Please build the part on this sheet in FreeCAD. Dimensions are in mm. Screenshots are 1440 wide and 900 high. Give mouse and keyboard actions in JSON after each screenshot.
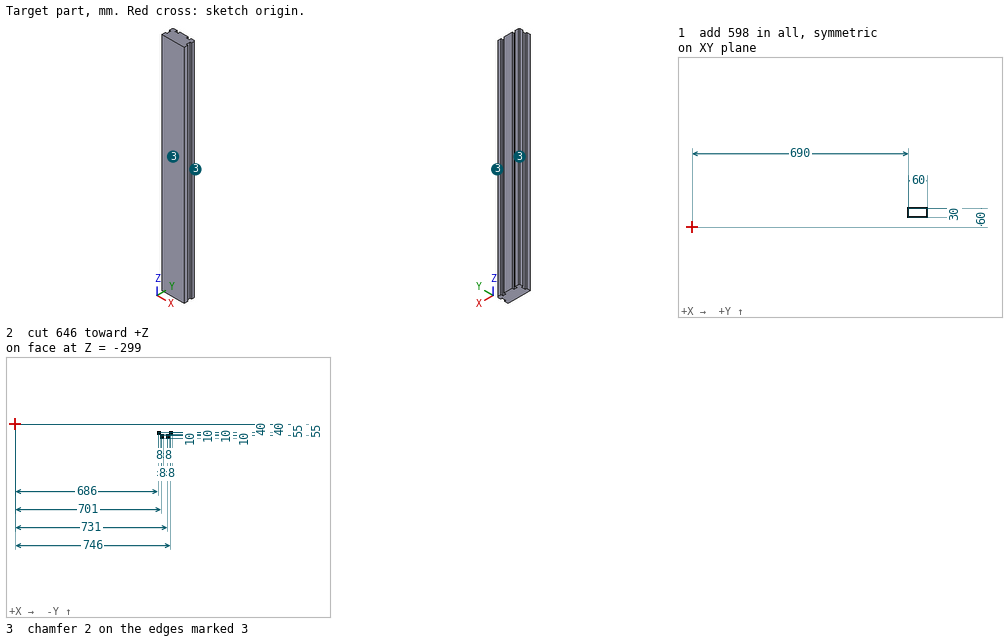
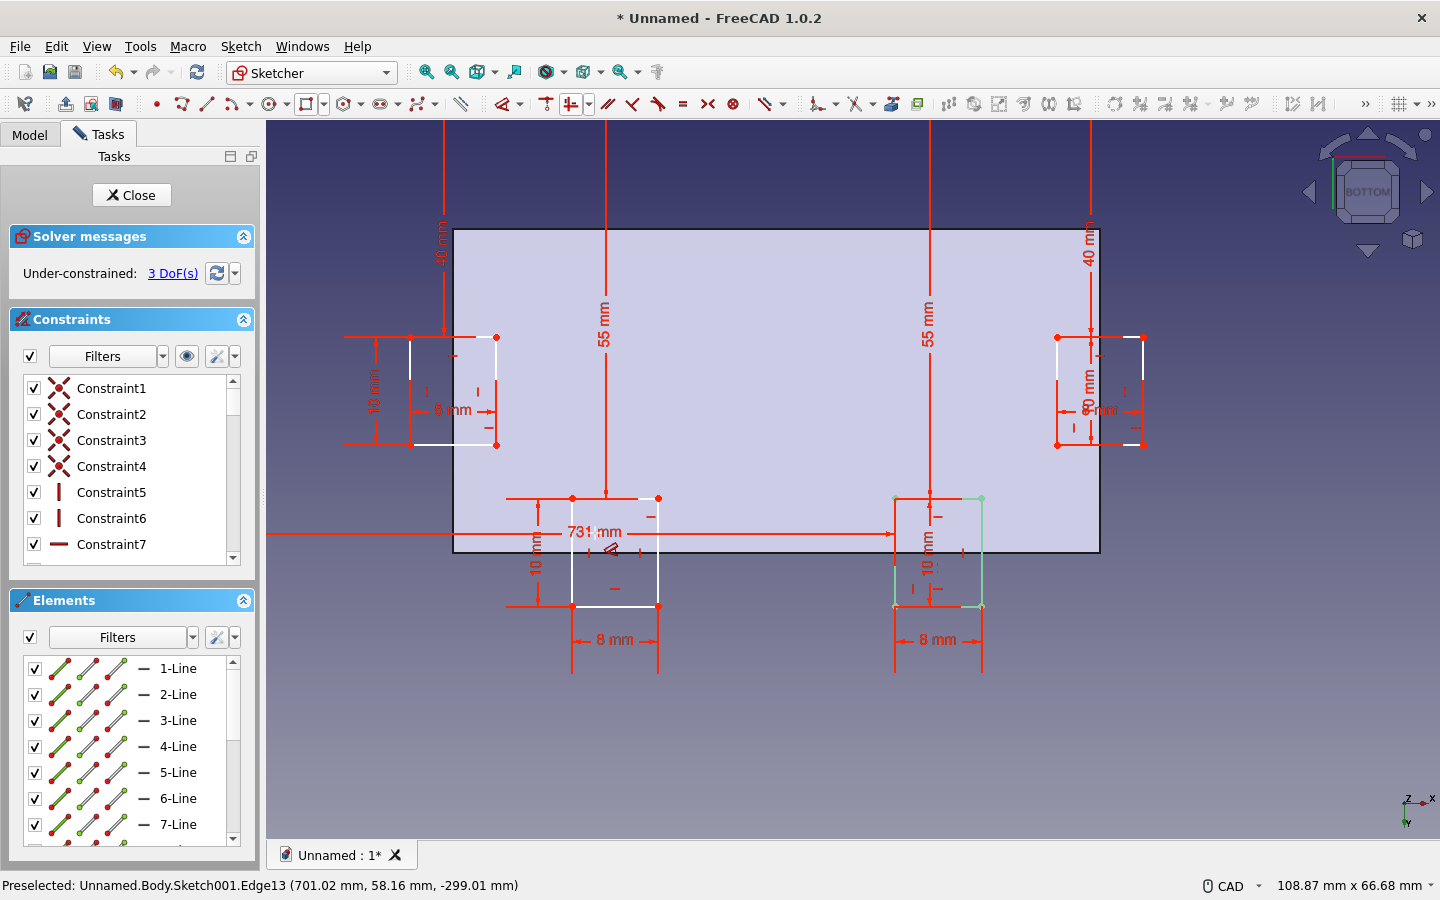
{"action": "left_click", "coordinate": [1057, 337]}
{"action": "left_click", "coordinate": [676, 371]}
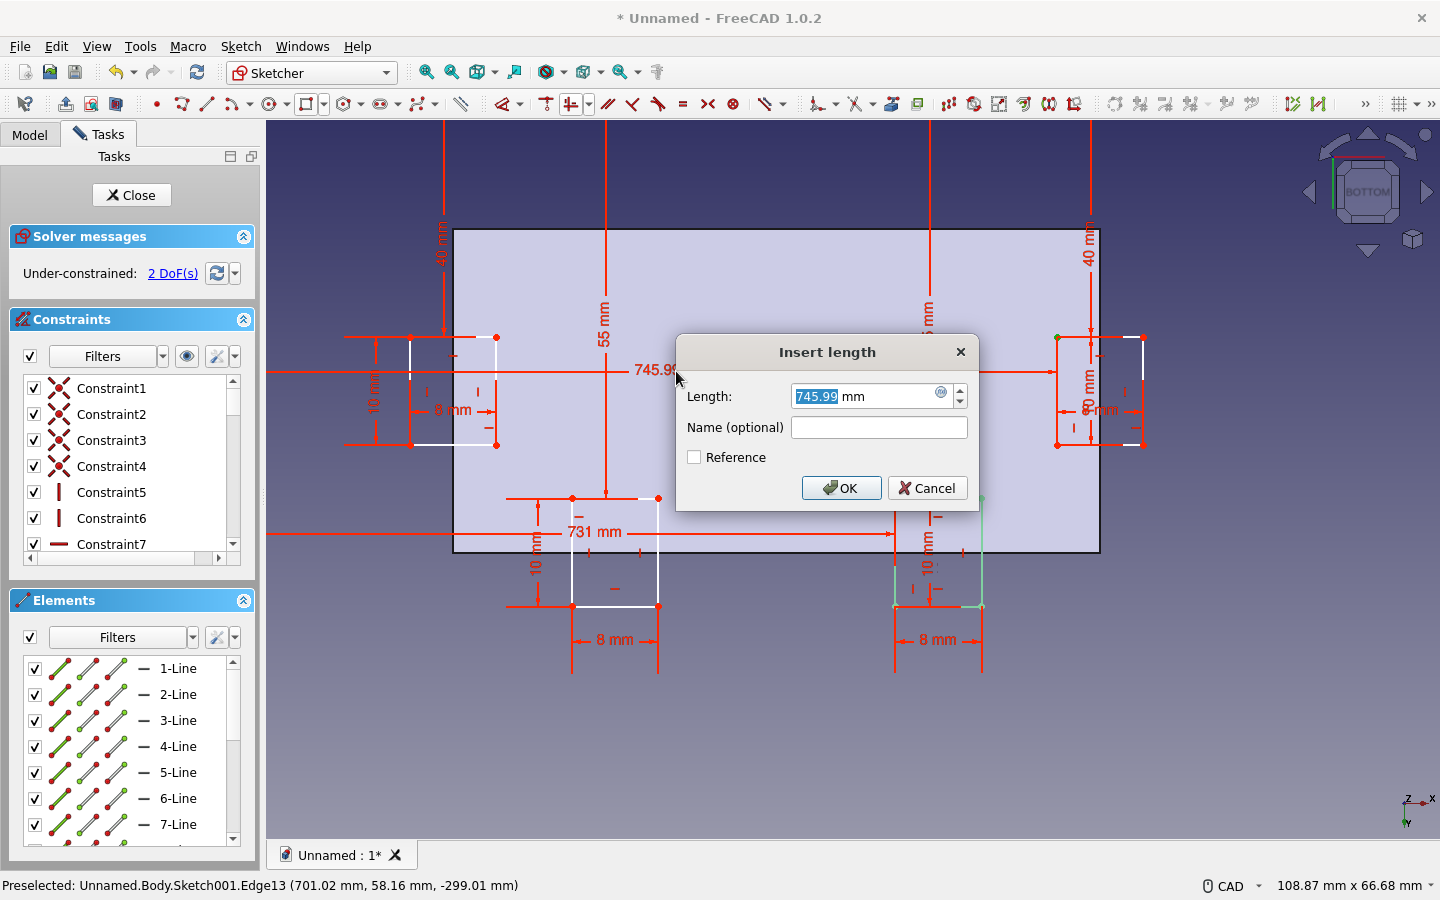
{"action": "type", "text": "746"}
{"action": "key", "text": "Return"}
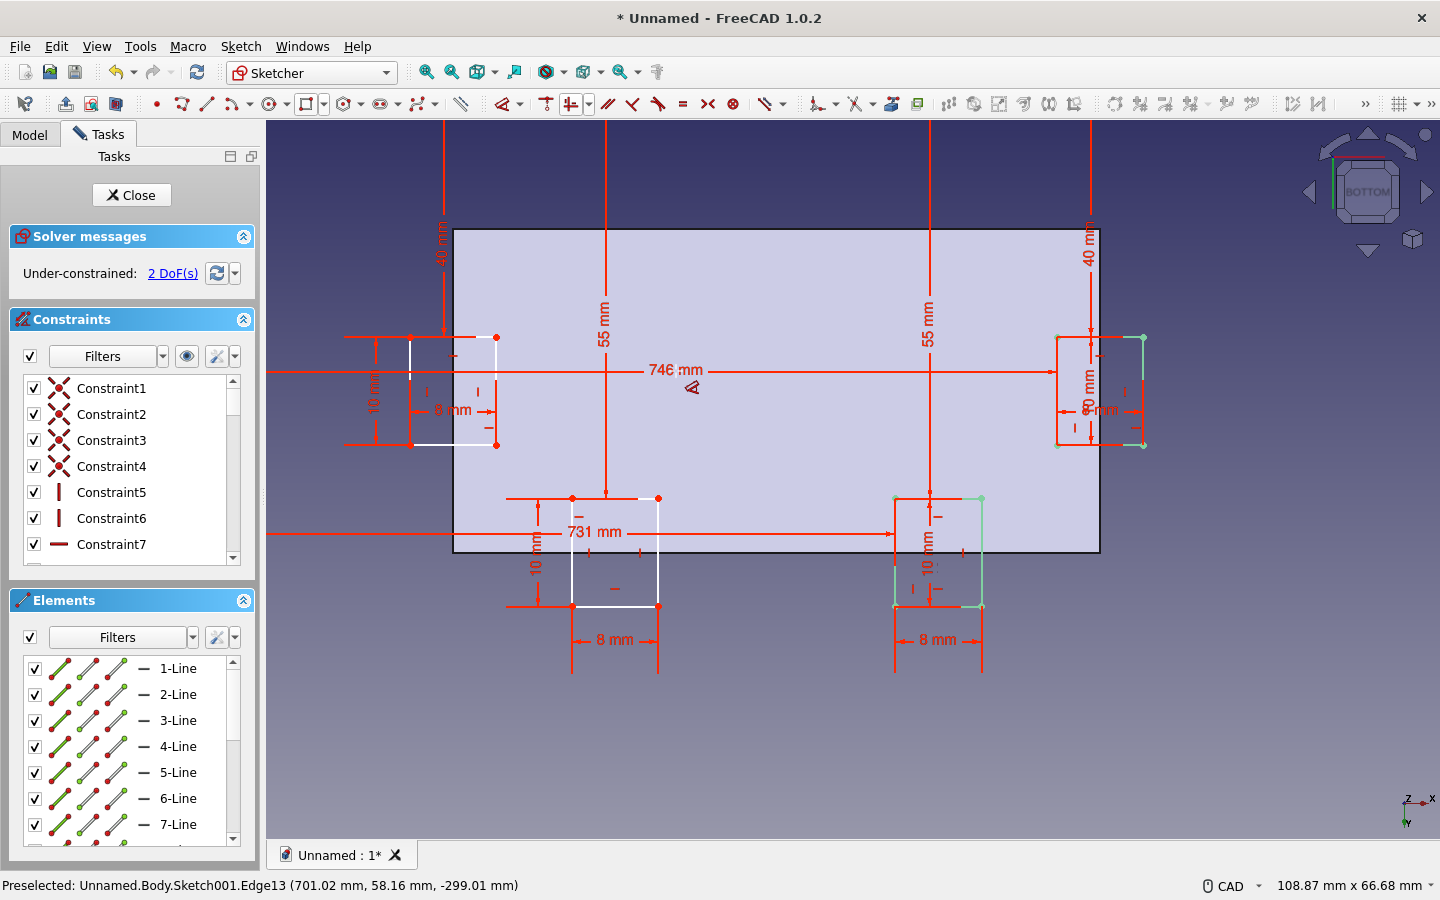
{"action": "left_click", "coordinate": [410, 337]}
{"action": "left_click", "coordinate": [352, 371]}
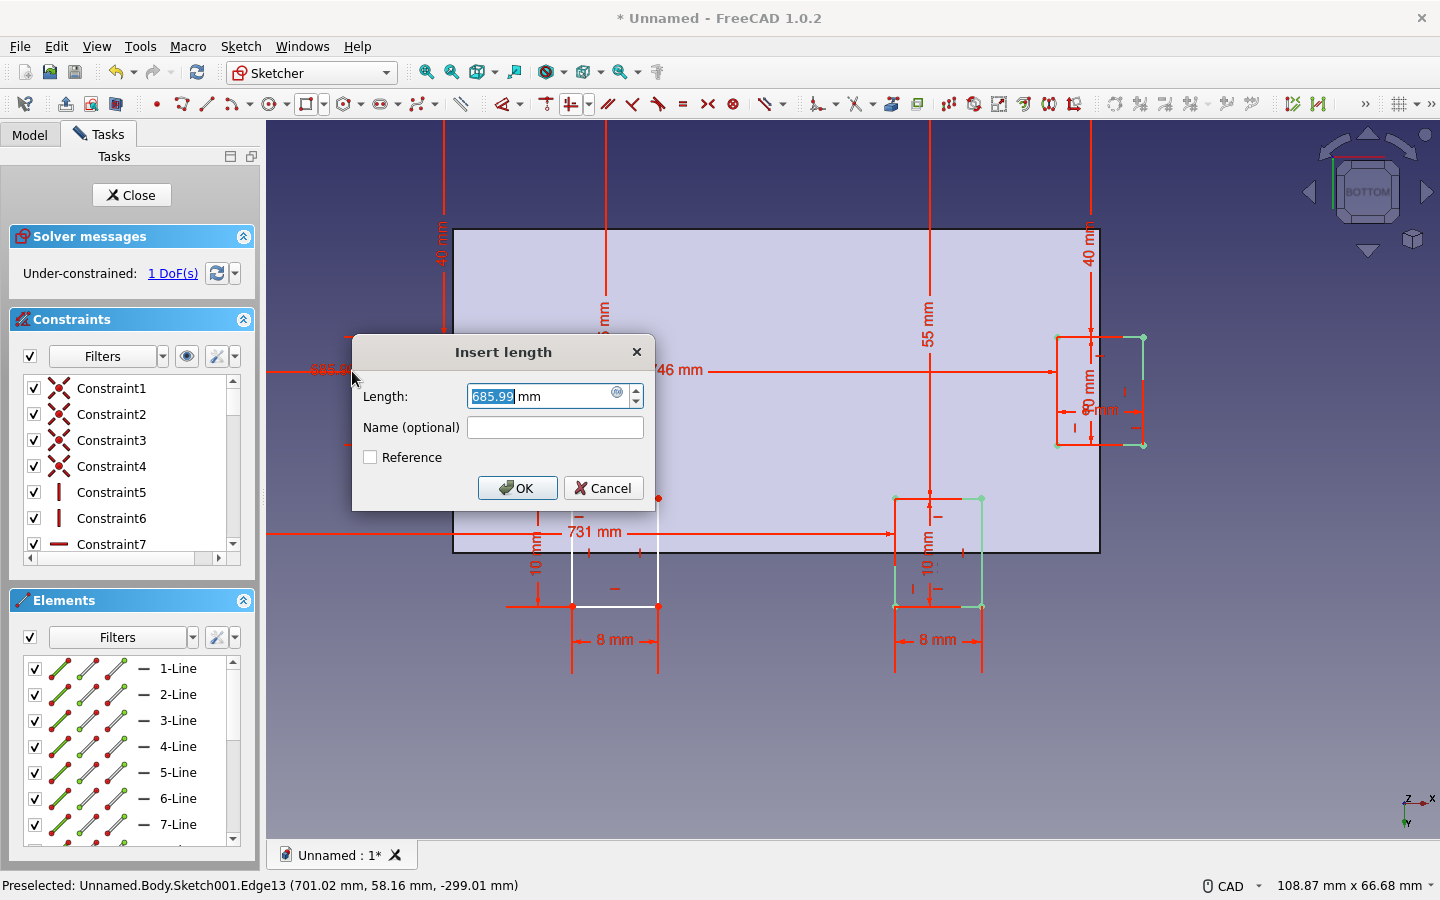
{"action": "type", "text": "686"}
{"action": "key", "text": "Return"}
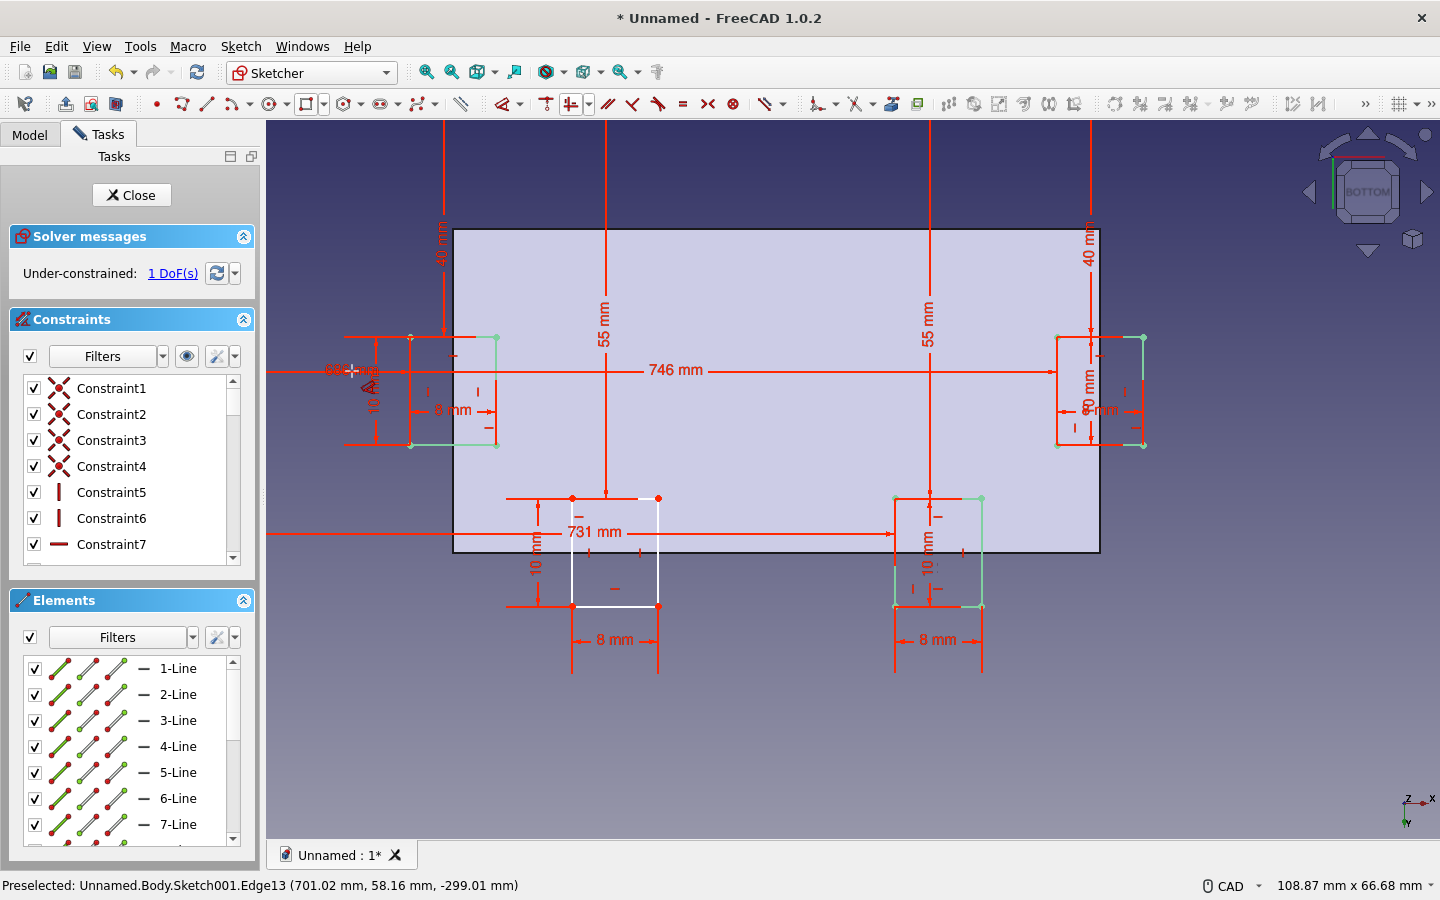
{"action": "left_click", "coordinate": [572, 499]}
{"action": "left_click", "coordinate": [433, 533]}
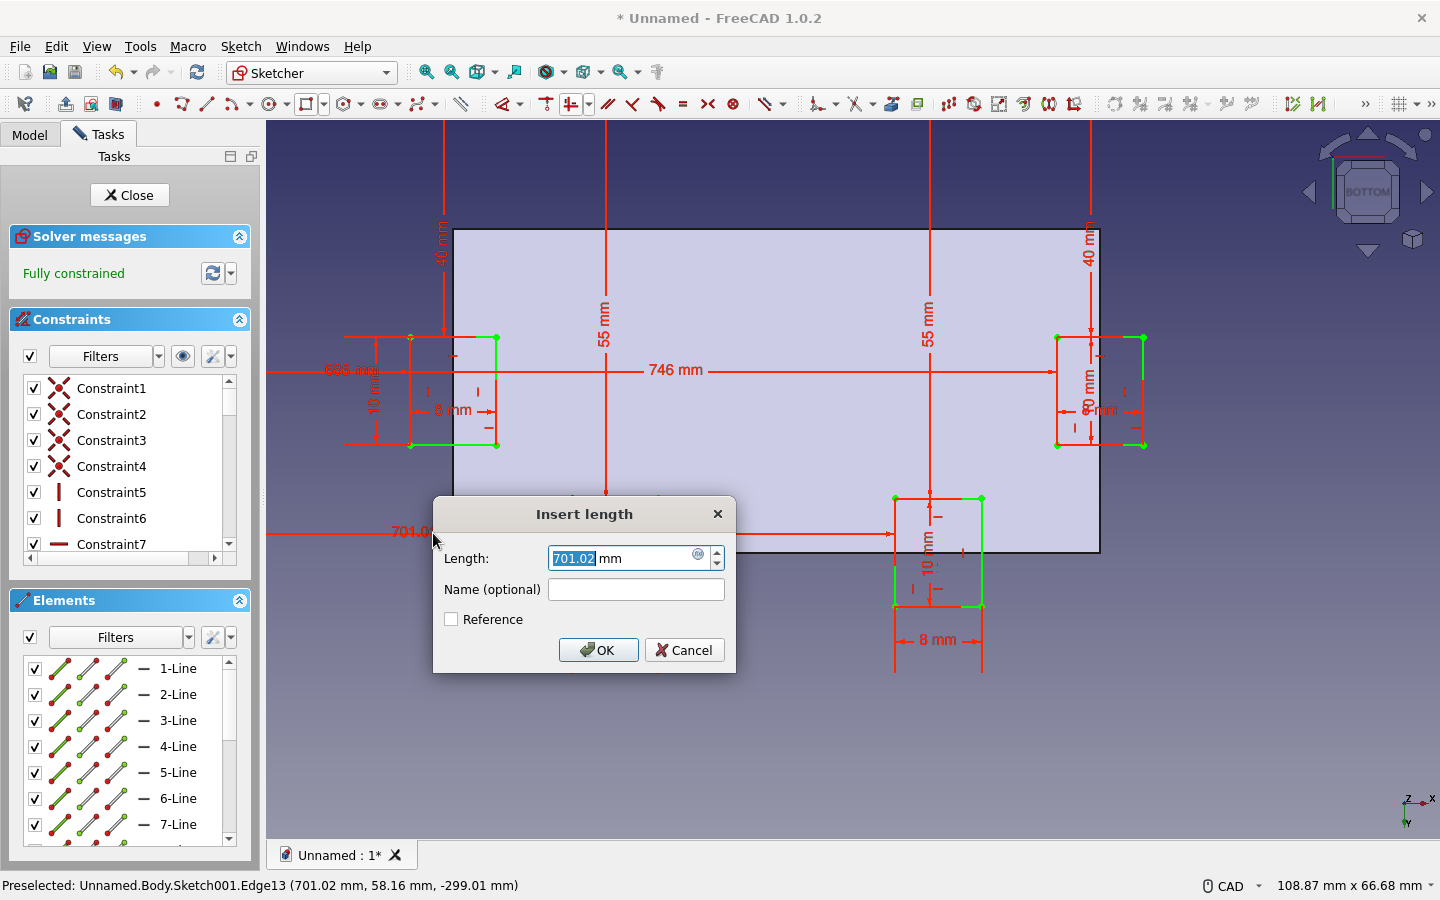
{"action": "type", "text": "701"}
{"action": "key", "text": "Return"}
{"action": "key", "text": "Escape"}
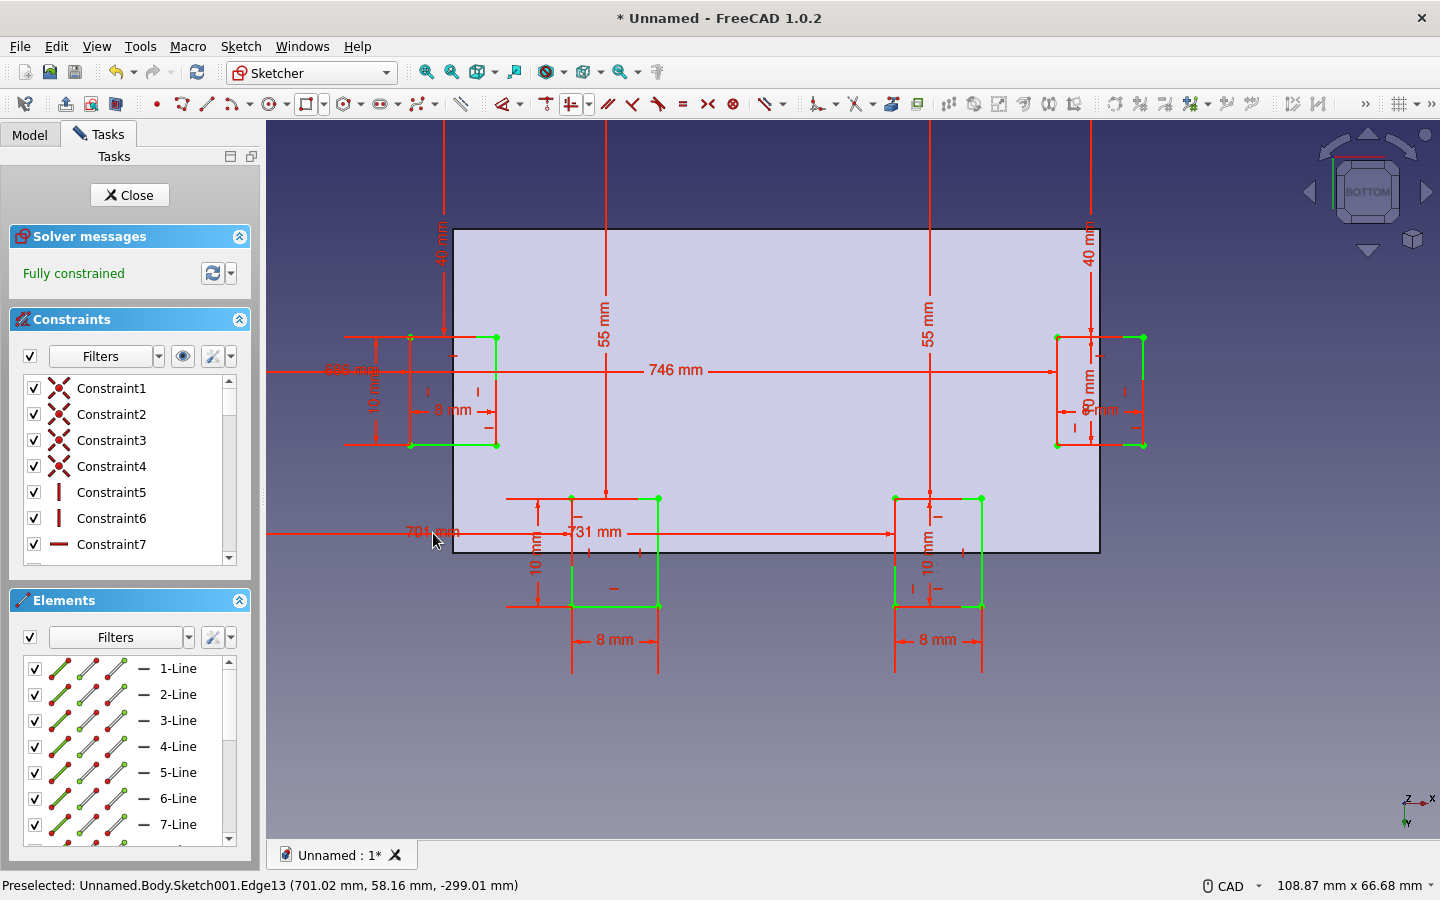
{"action": "left_click", "coordinate": [130, 195]}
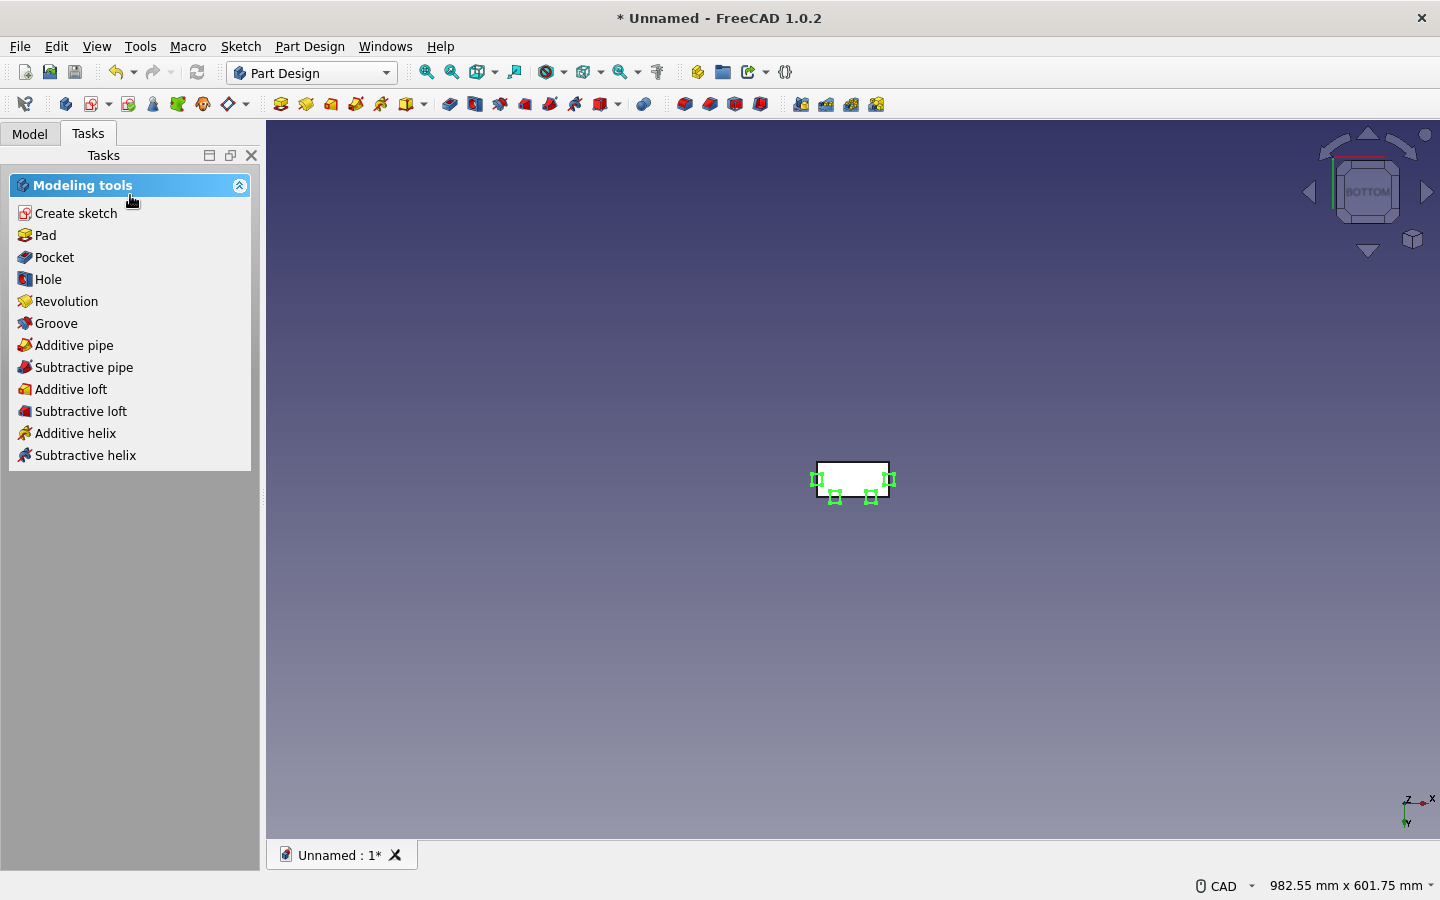
{"action": "left_click", "coordinate": [450, 104]}